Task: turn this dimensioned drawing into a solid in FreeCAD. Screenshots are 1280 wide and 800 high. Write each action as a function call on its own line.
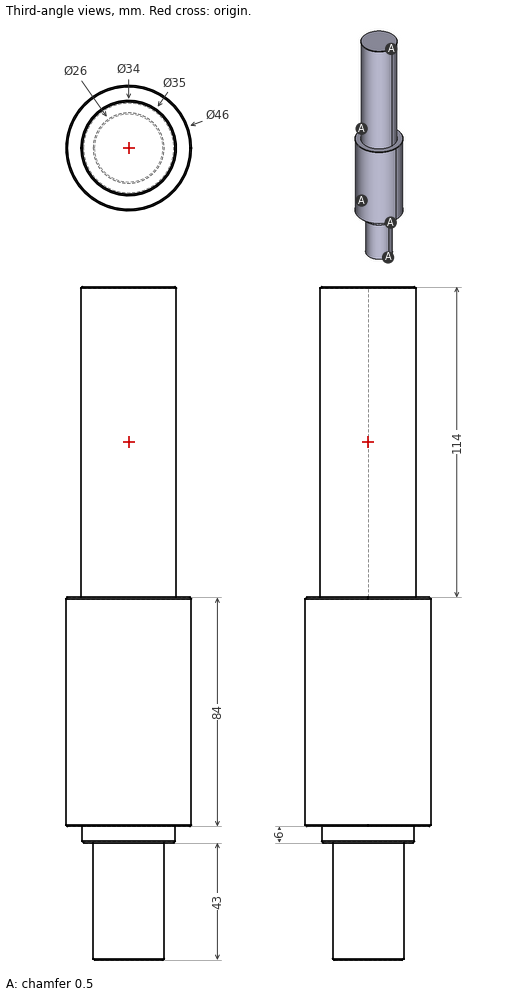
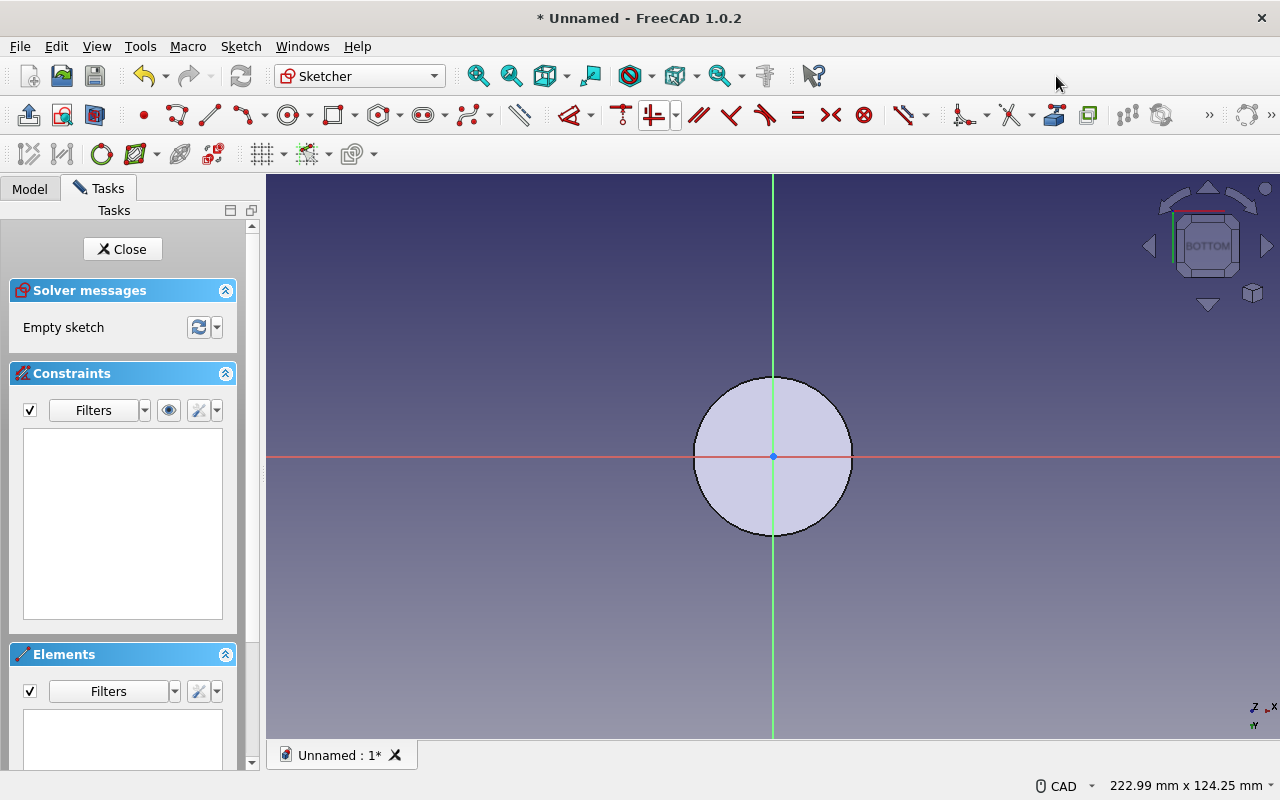
scroll(856, 456, up, 3)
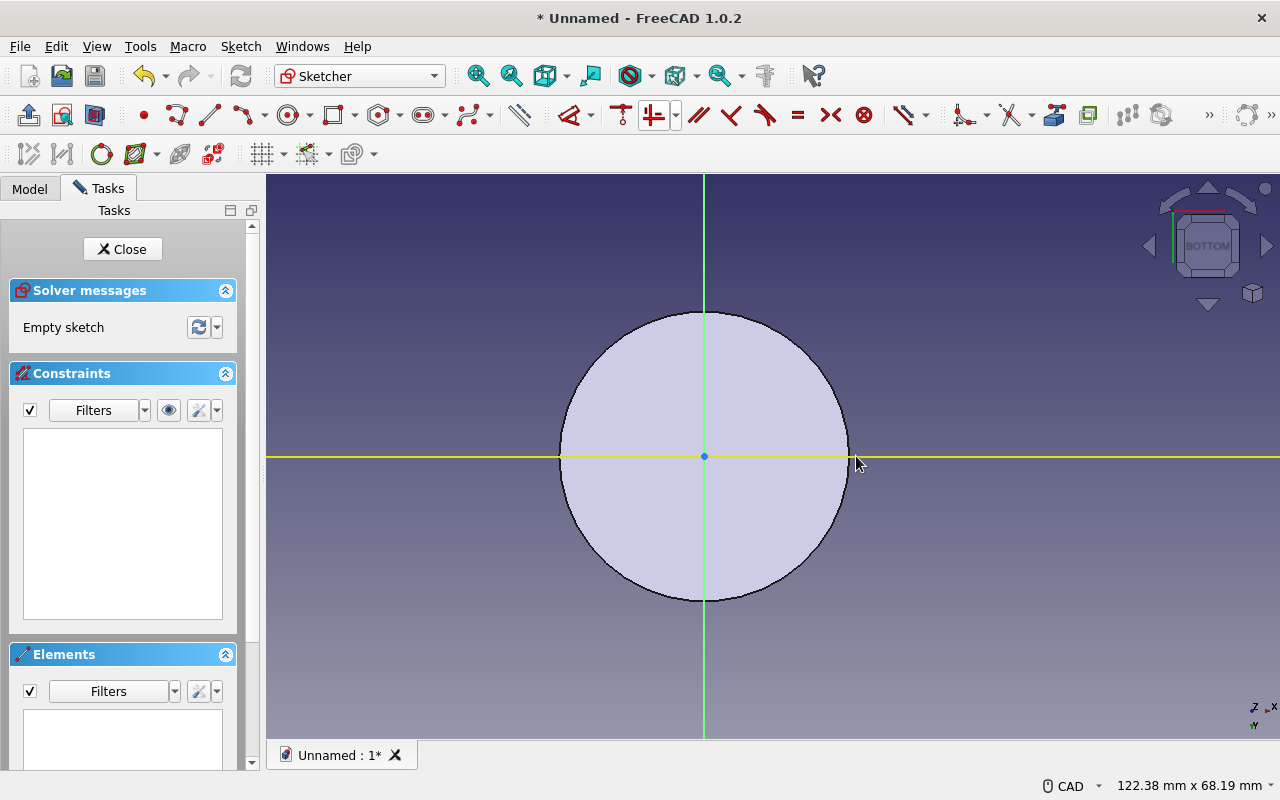
click(288, 116)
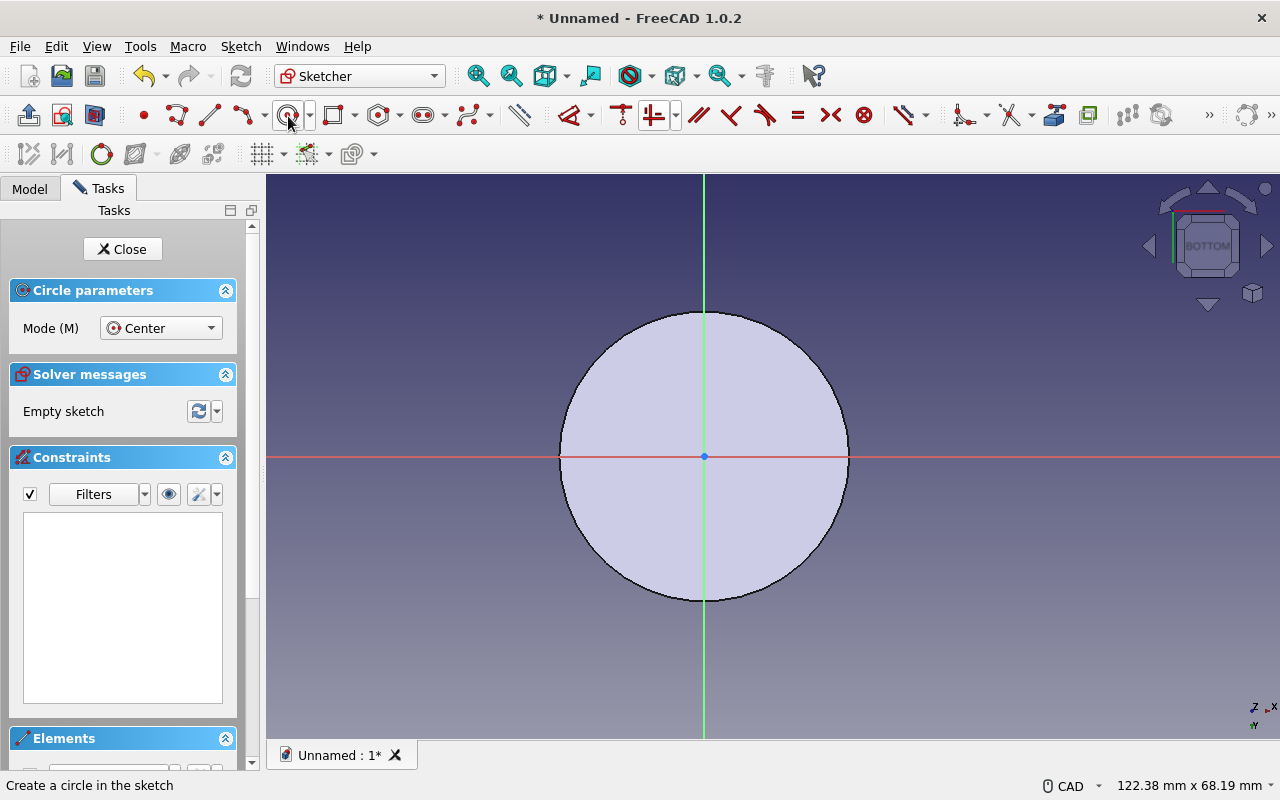
click(704, 456)
click(839, 322)
key(Escape)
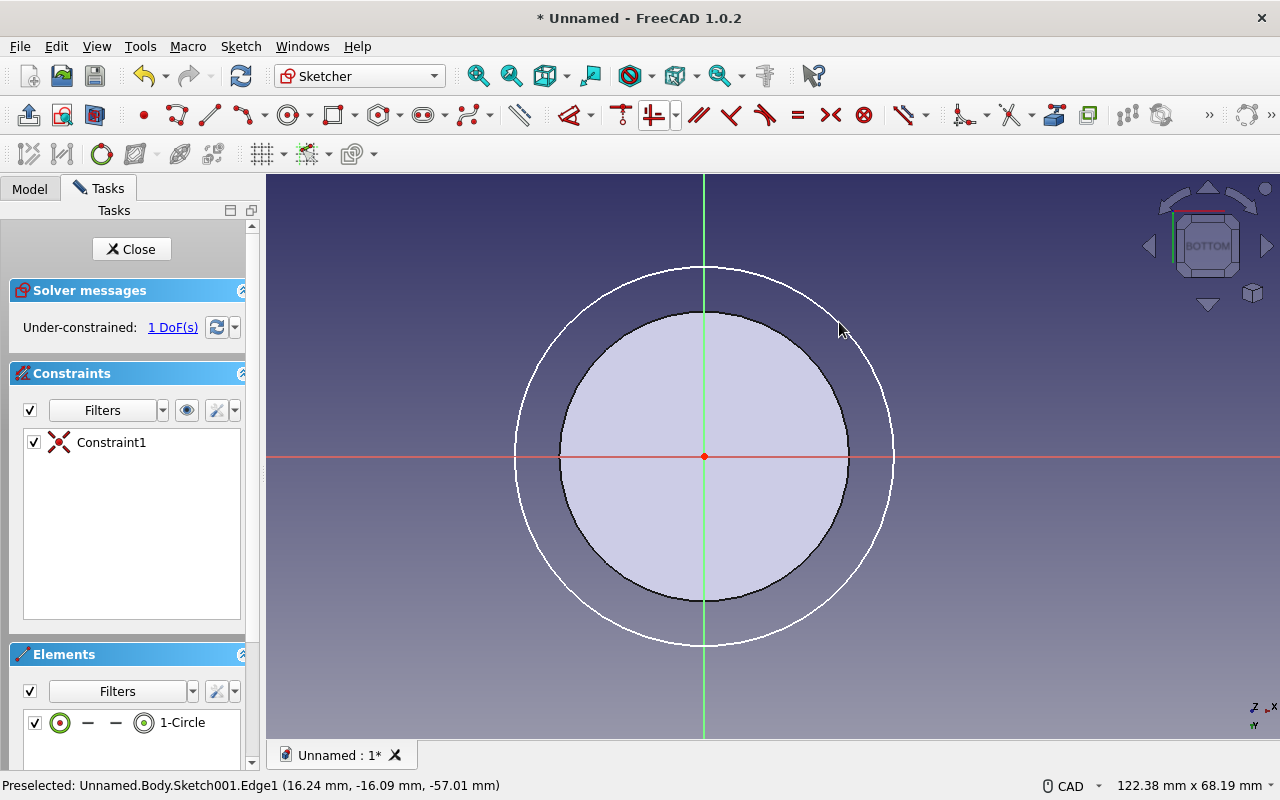
key(d)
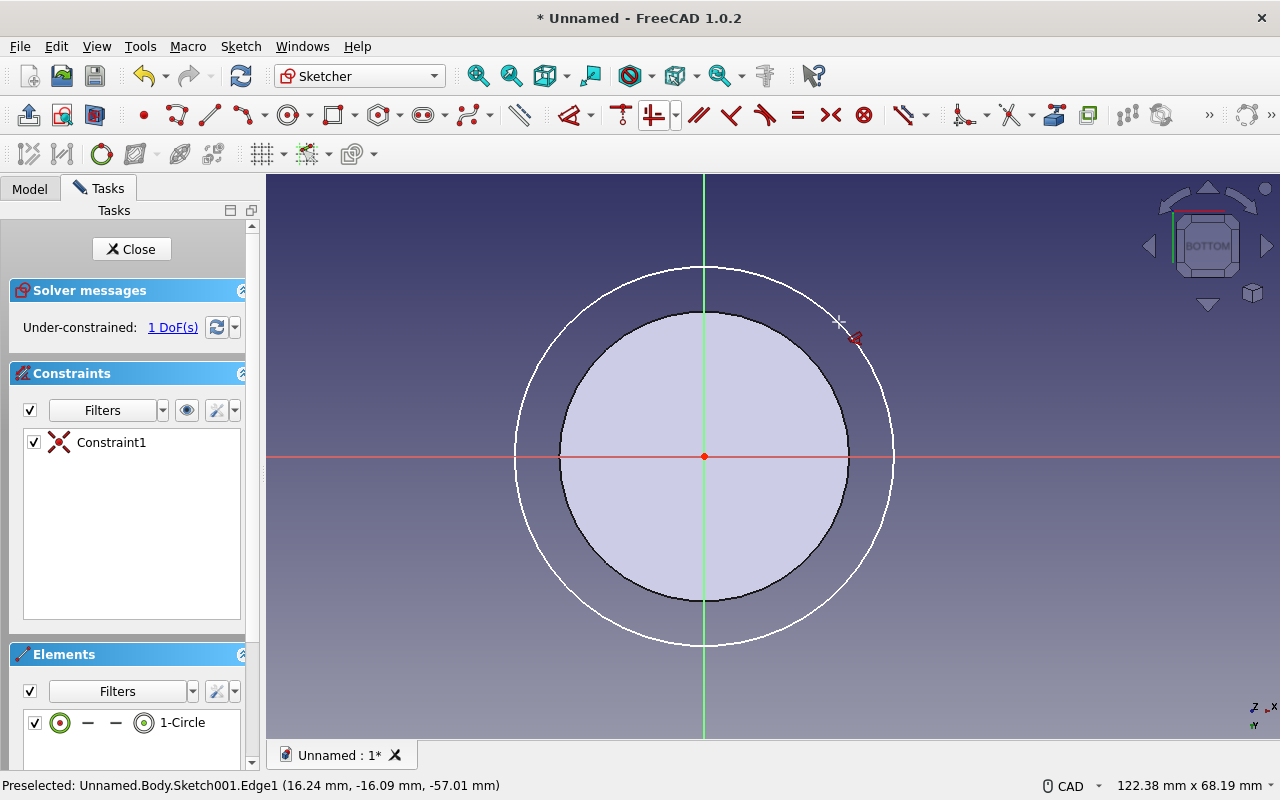
click(838, 322)
click(861, 299)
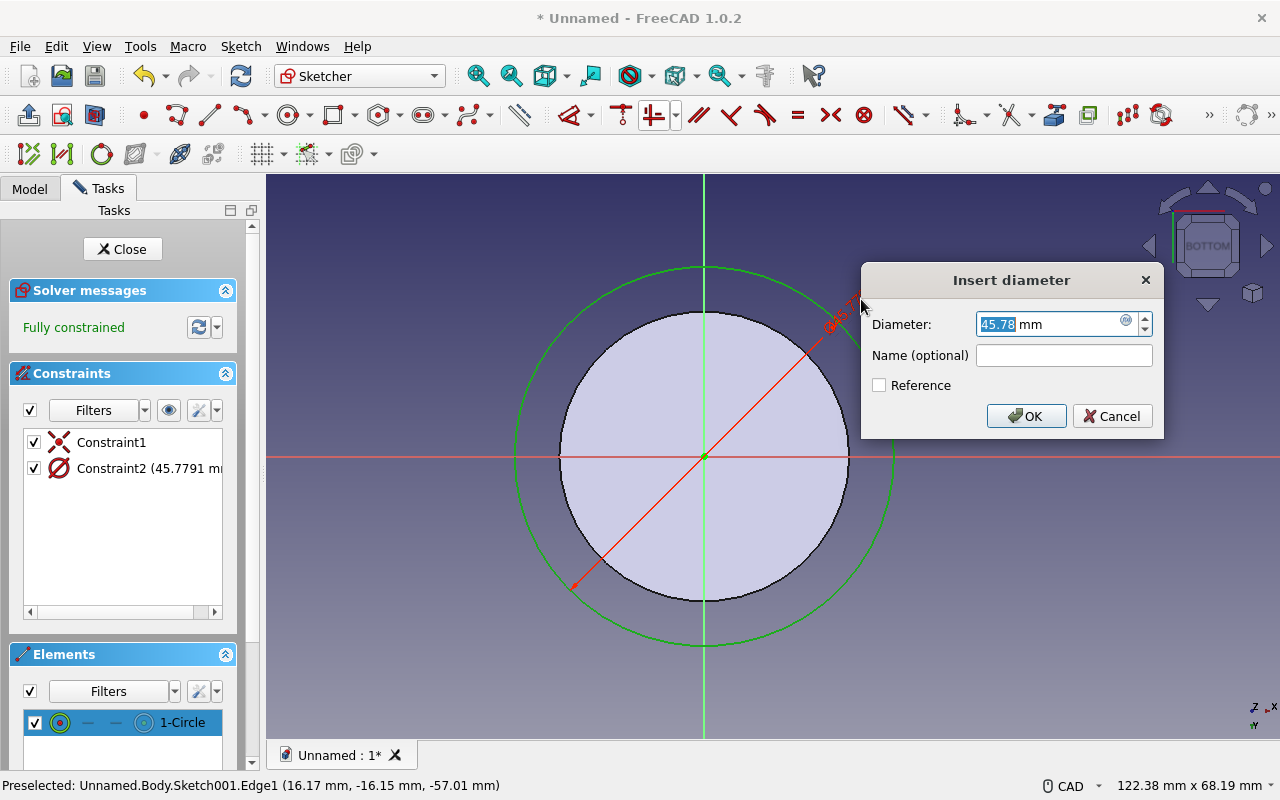
text(46)
key(Return)
key(Escape)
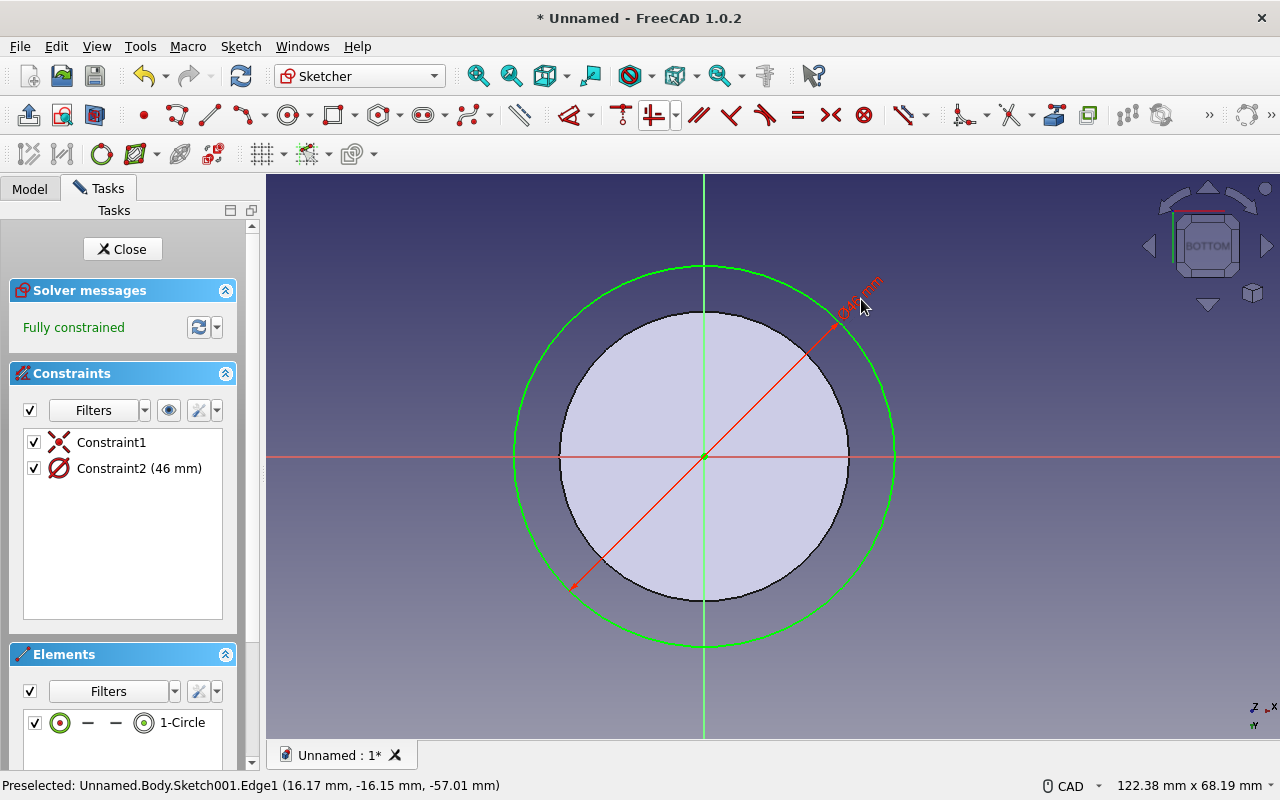
click(123, 249)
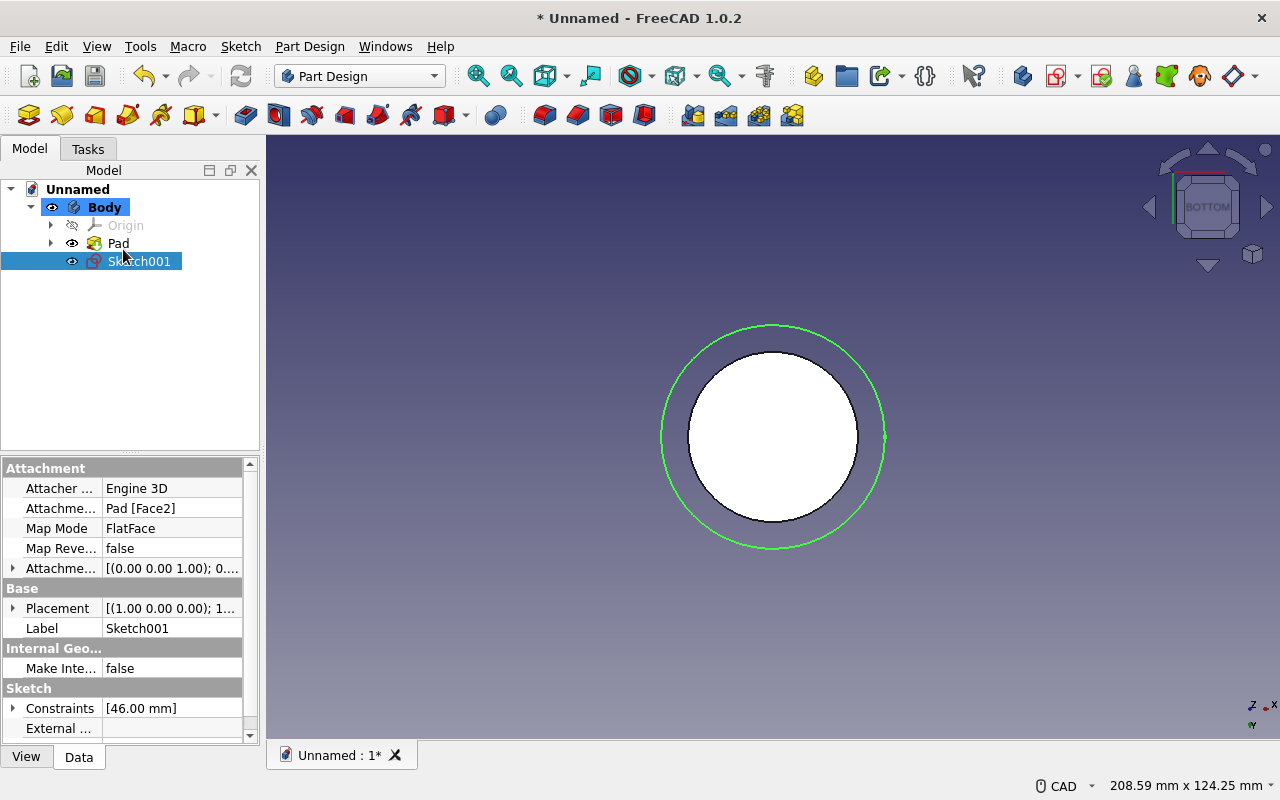
click(29, 116)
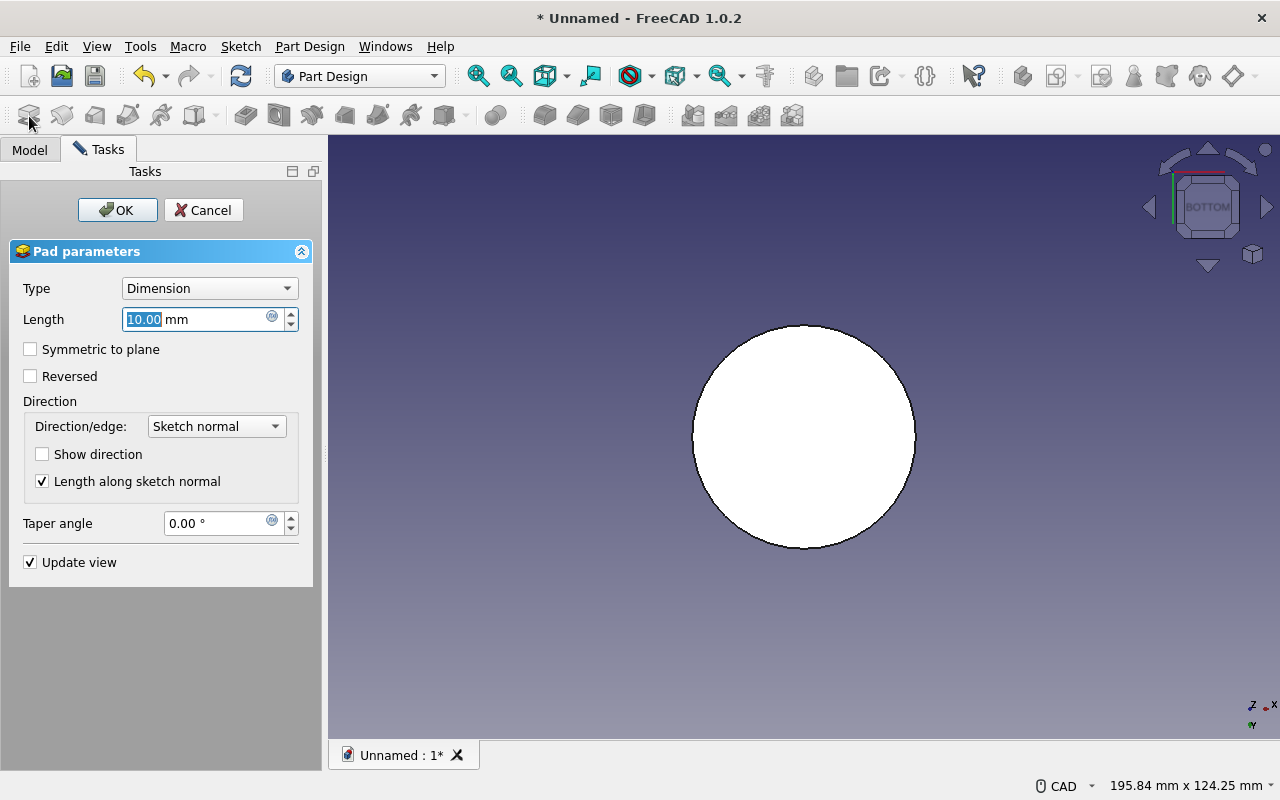
text(84)
key(Tab)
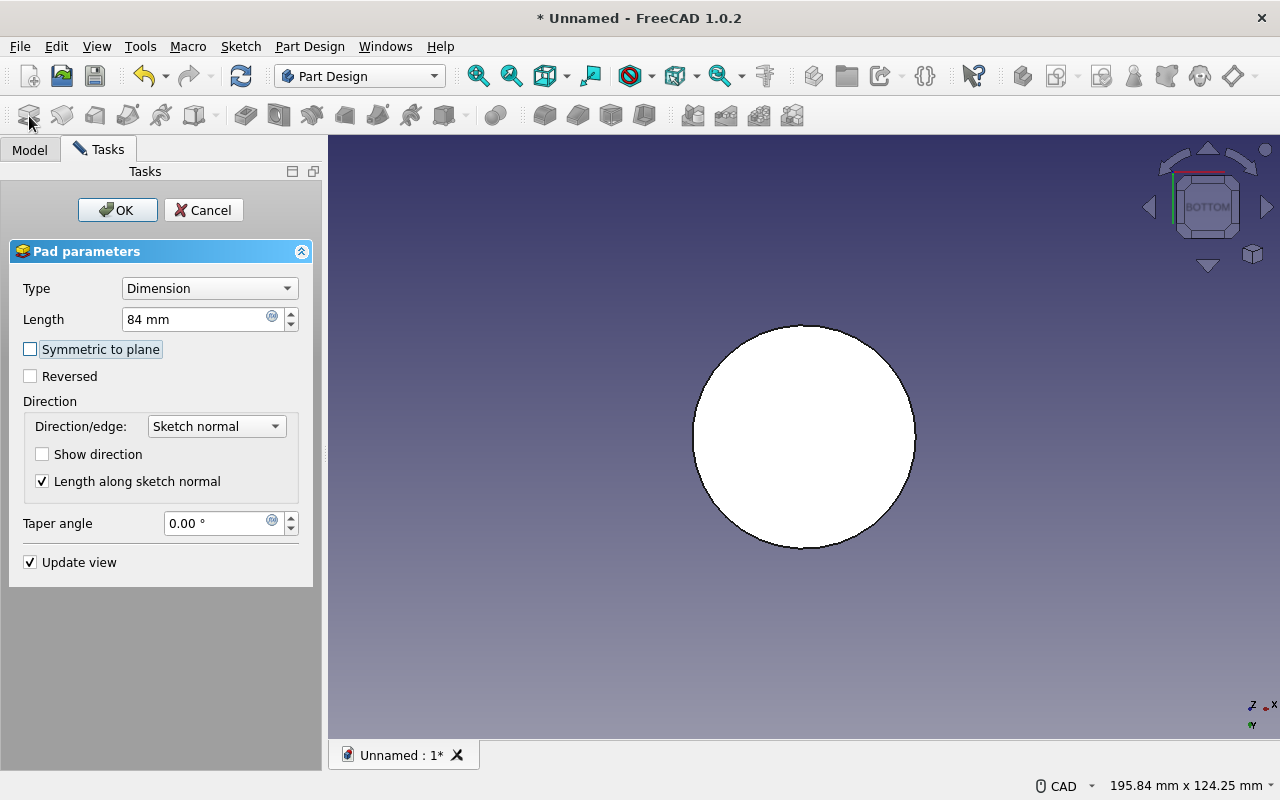
click(118, 210)